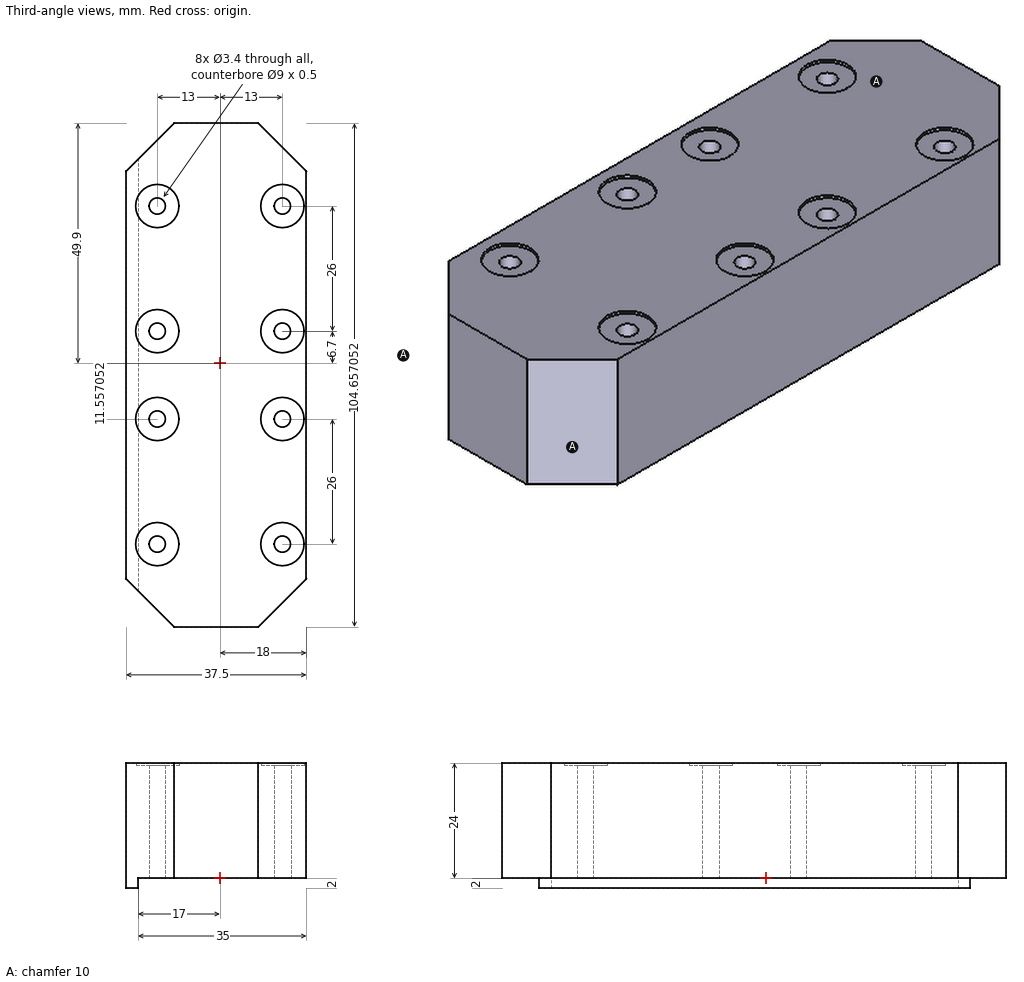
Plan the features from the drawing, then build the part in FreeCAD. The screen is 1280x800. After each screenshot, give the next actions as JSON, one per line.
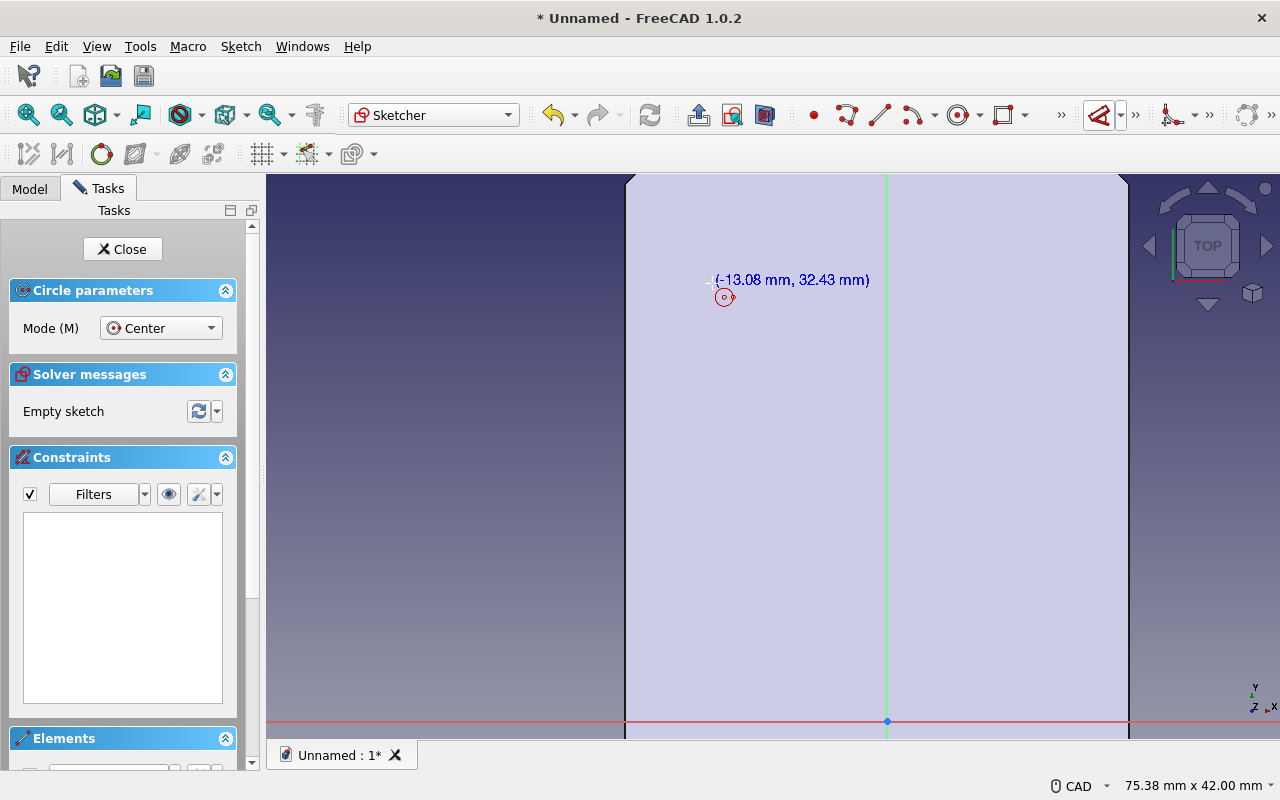
{"action": "left_click", "coordinate": [712, 282]}
{"action": "mouse_move", "coordinate": [728, 266]}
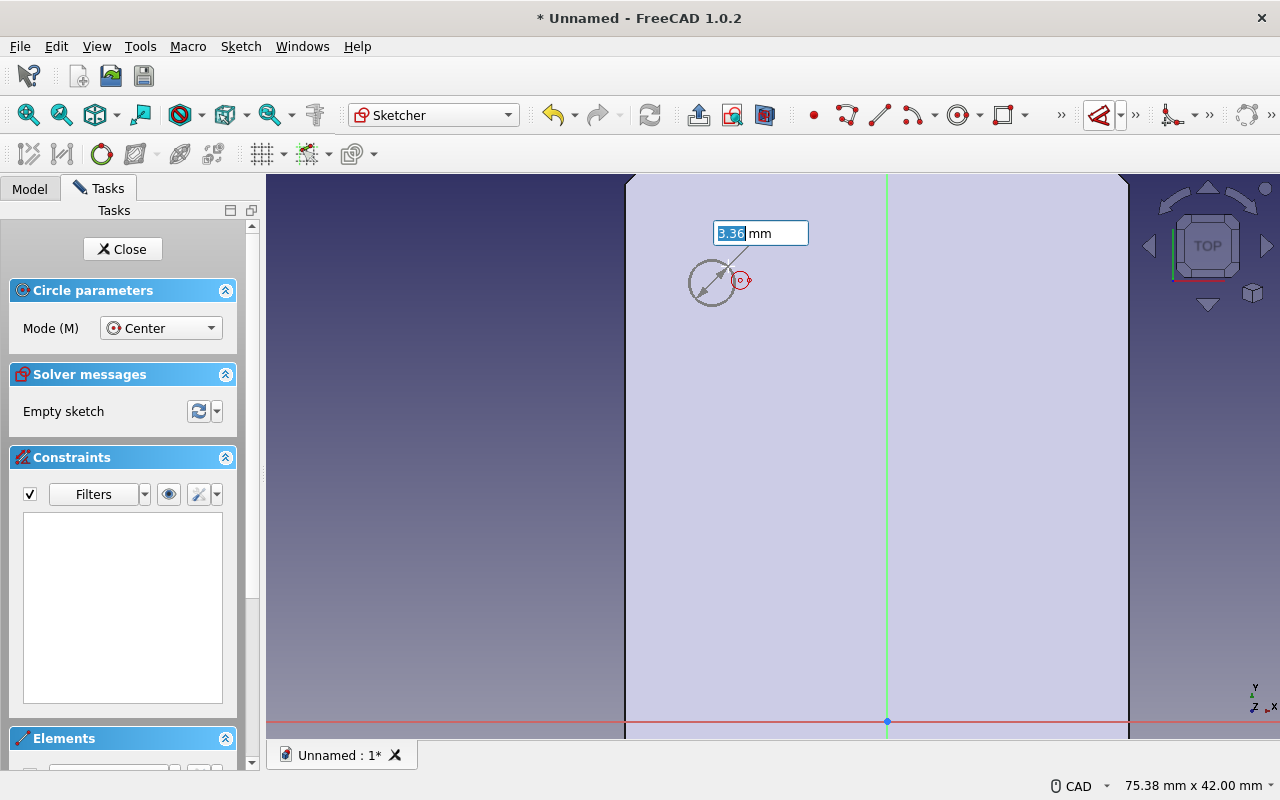
{"action": "type", "text": "3.4"}
{"action": "key", "text": "Return"}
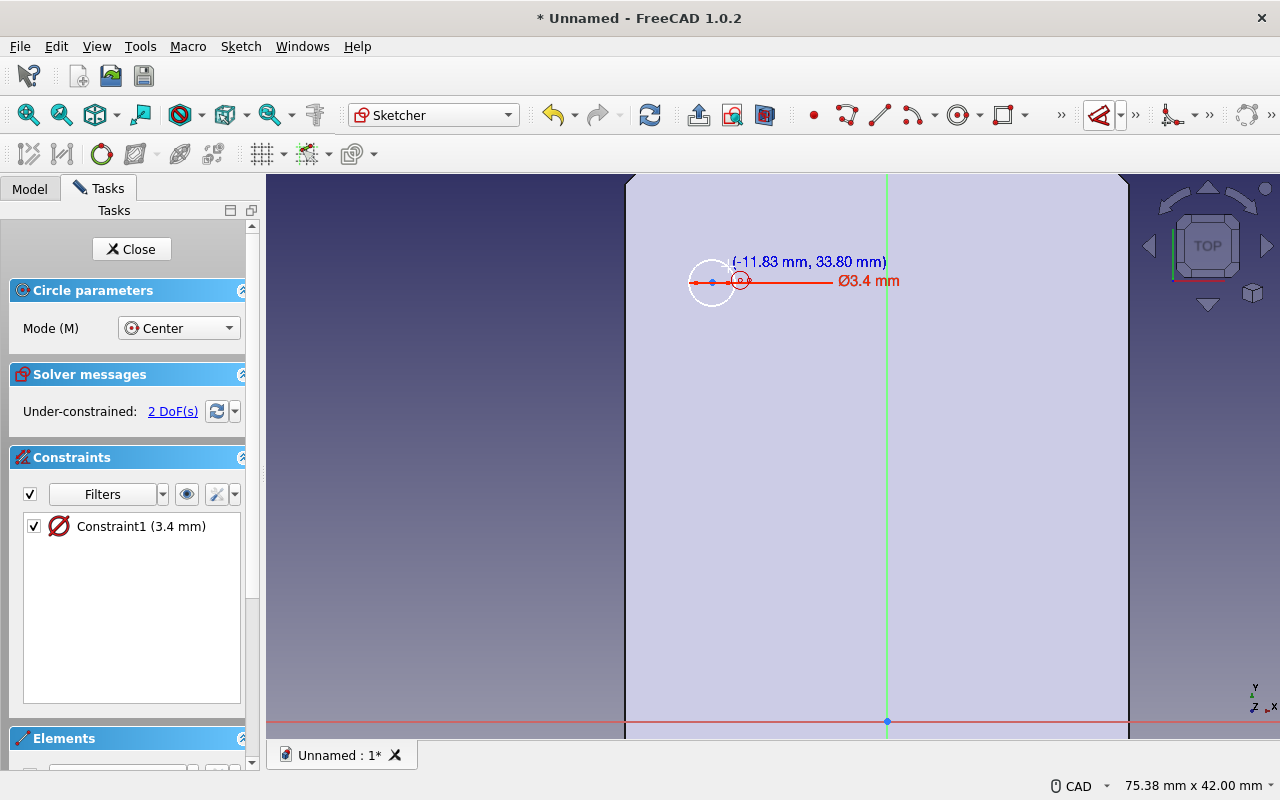
{"action": "left_click", "coordinate": [1062, 282]}
{"action": "mouse_move", "coordinate": [1078, 266]}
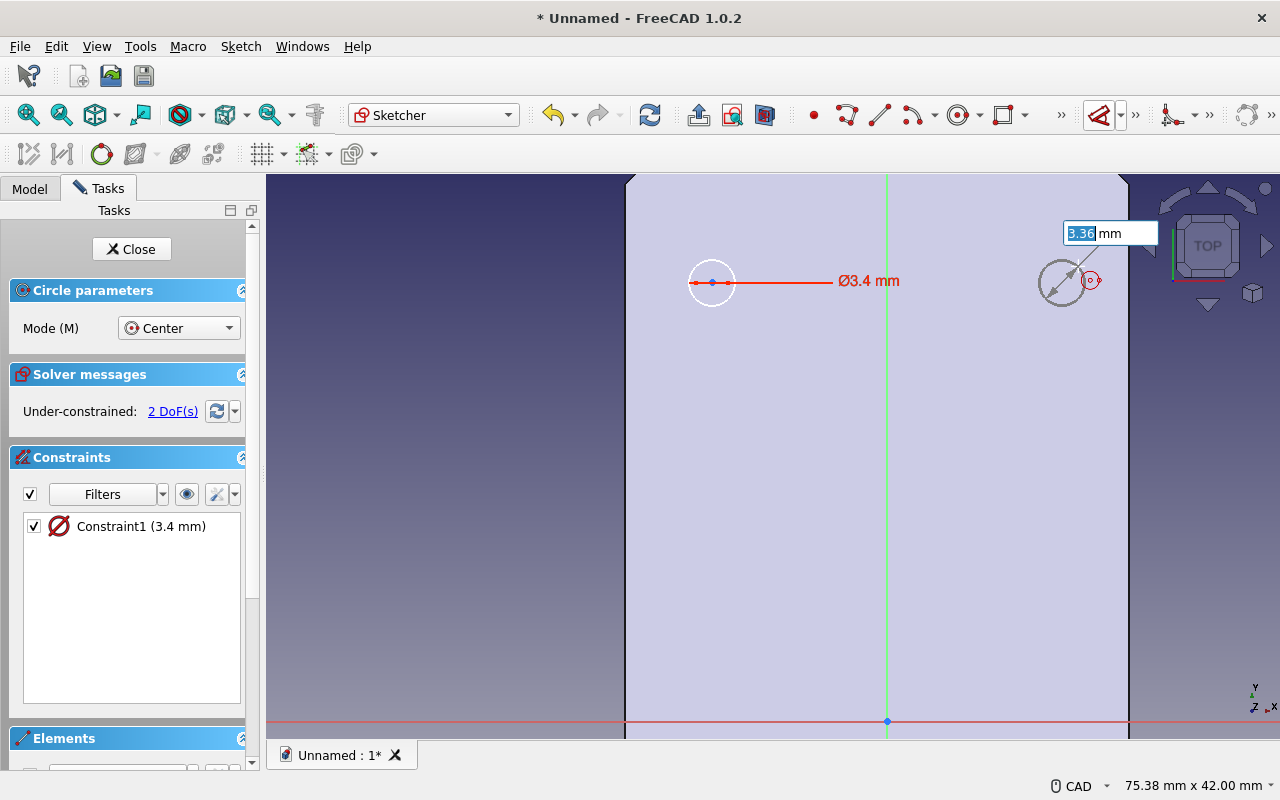
{"action": "type", "text": "3.4"}
{"action": "key", "text": "Return"}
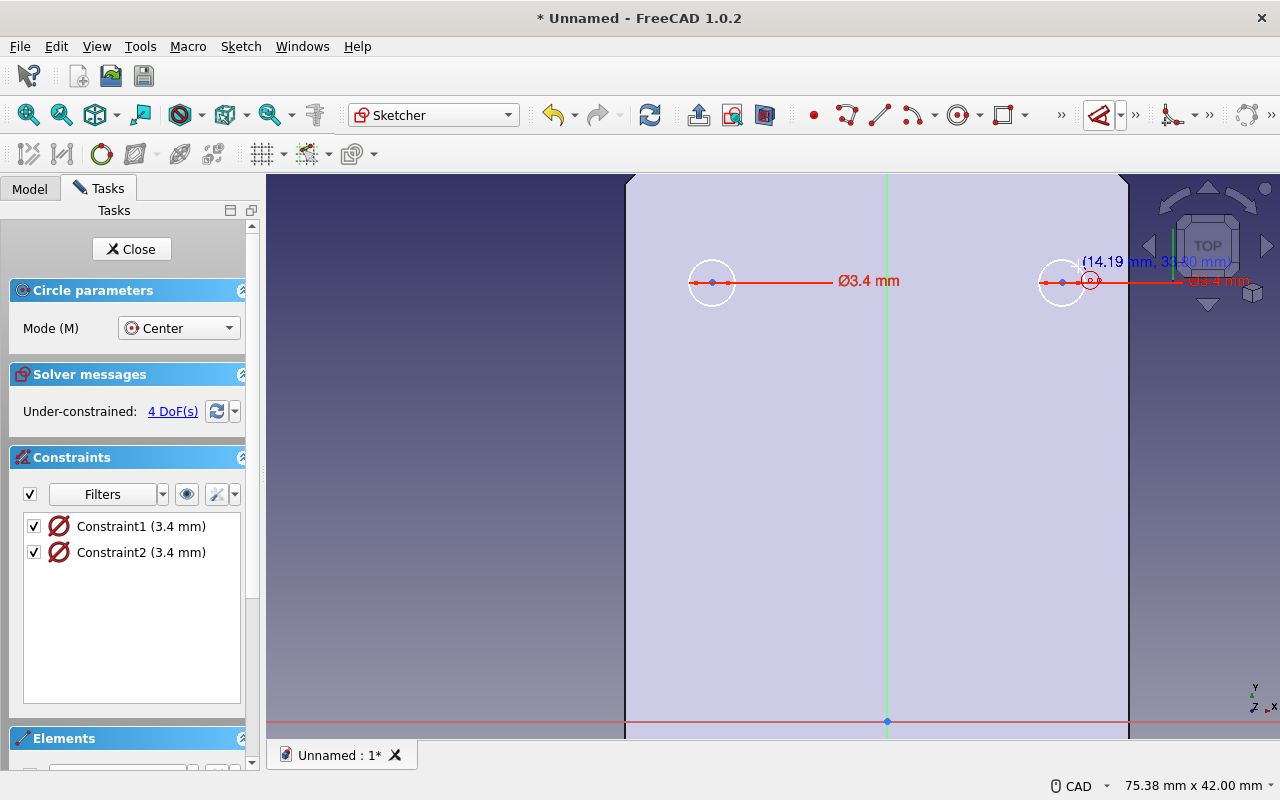
{"action": "left_click", "coordinate": [1062, 631]}
{"action": "mouse_move", "coordinate": [1078, 615]}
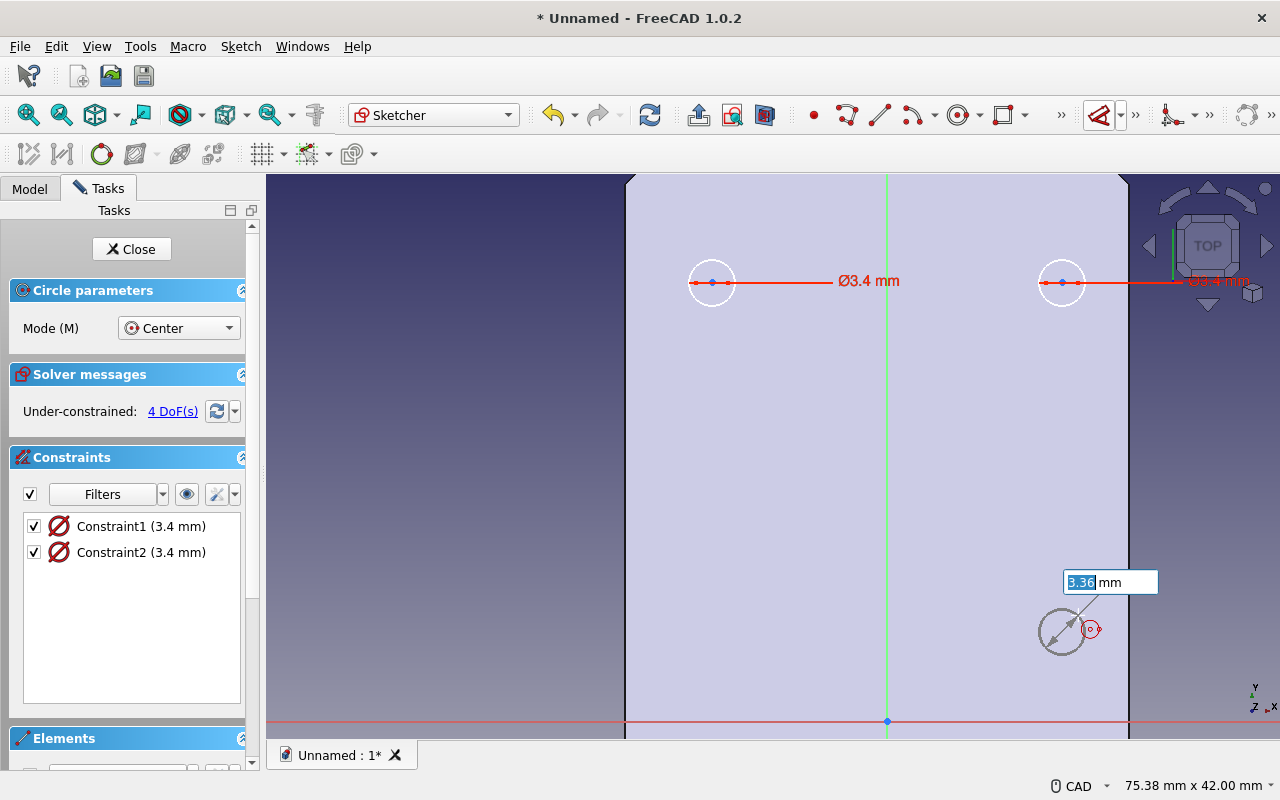
{"action": "type", "text": "3.4"}
{"action": "key", "text": "Return"}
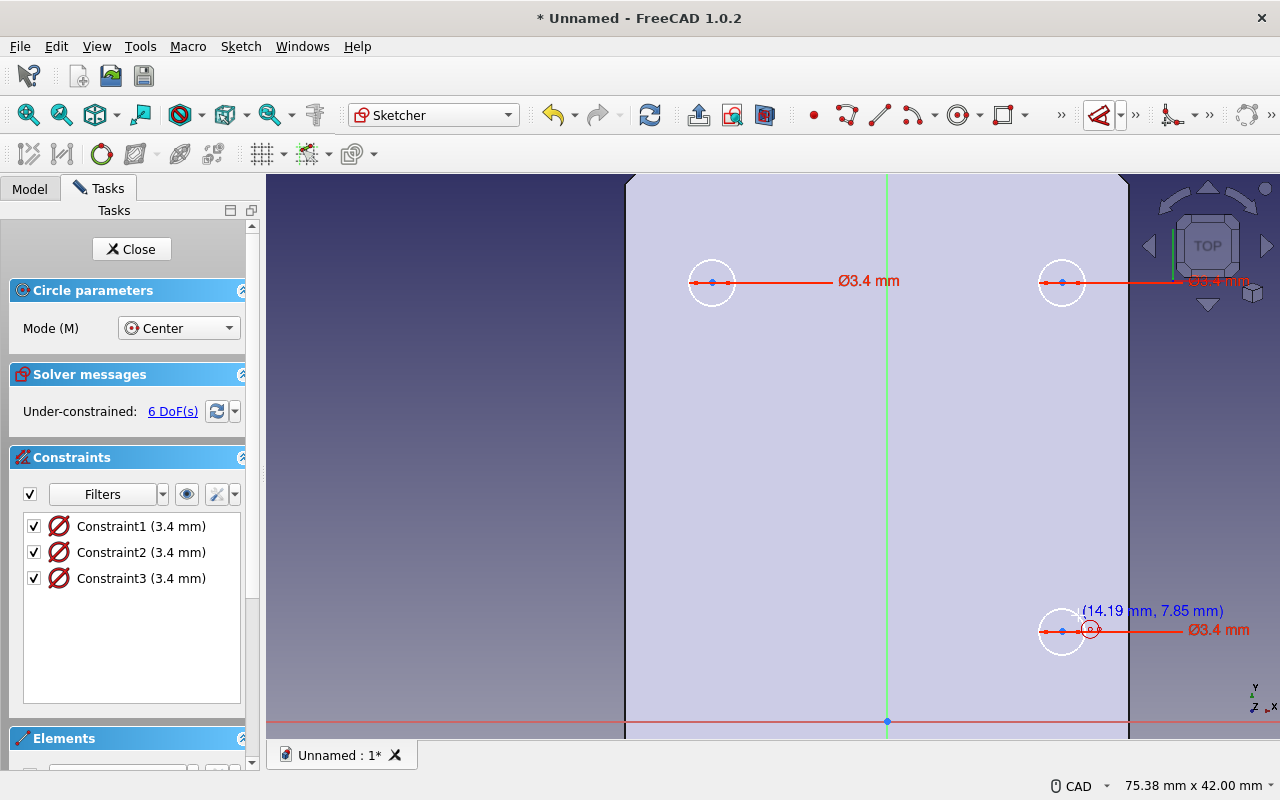
{"action": "left_click", "coordinate": [712, 631]}
{"action": "mouse_move", "coordinate": [728, 615]}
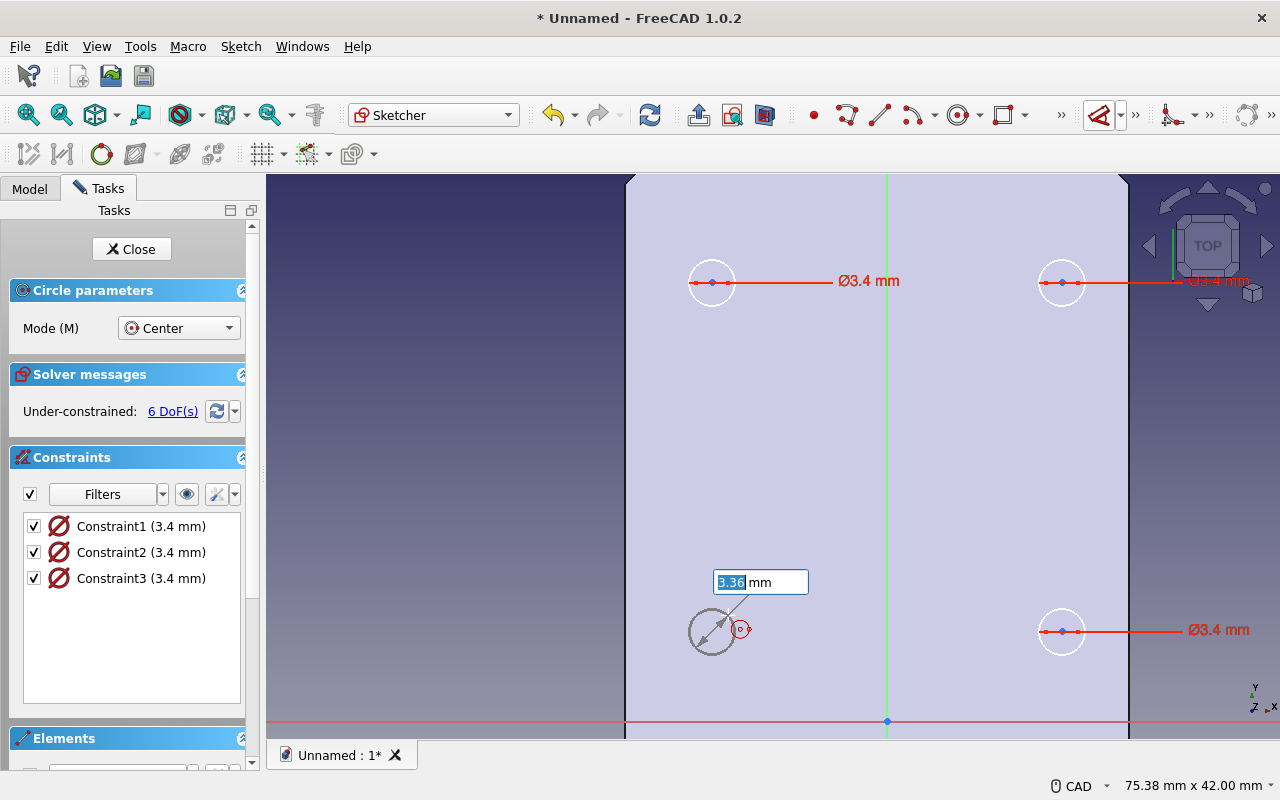
{"action": "type", "text": "3.4"}
{"action": "key", "text": "Return"}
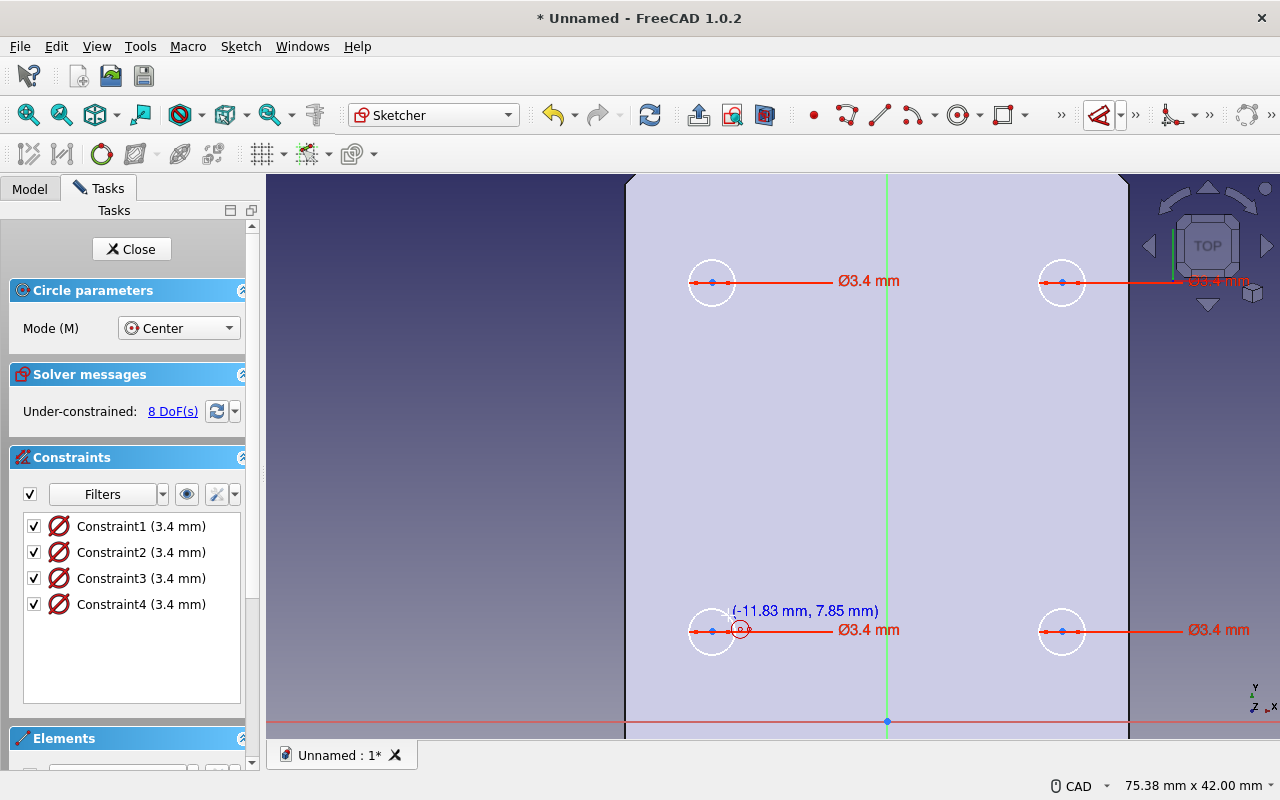
{"action": "scroll", "coordinate": [598, 283], "scroll_direction": "down", "scroll_amount": 5}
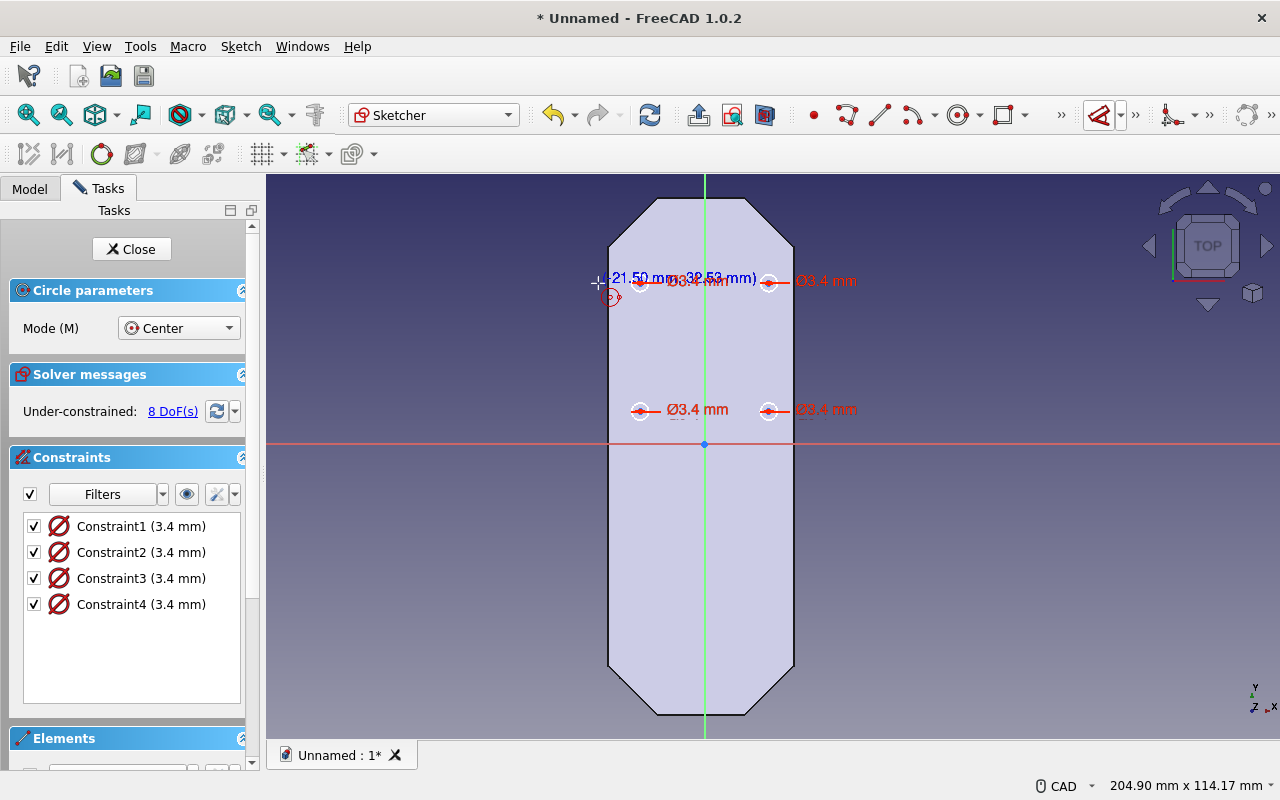
{"action": "scroll", "coordinate": [640, 502], "scroll_direction": "up", "scroll_amount": 5}